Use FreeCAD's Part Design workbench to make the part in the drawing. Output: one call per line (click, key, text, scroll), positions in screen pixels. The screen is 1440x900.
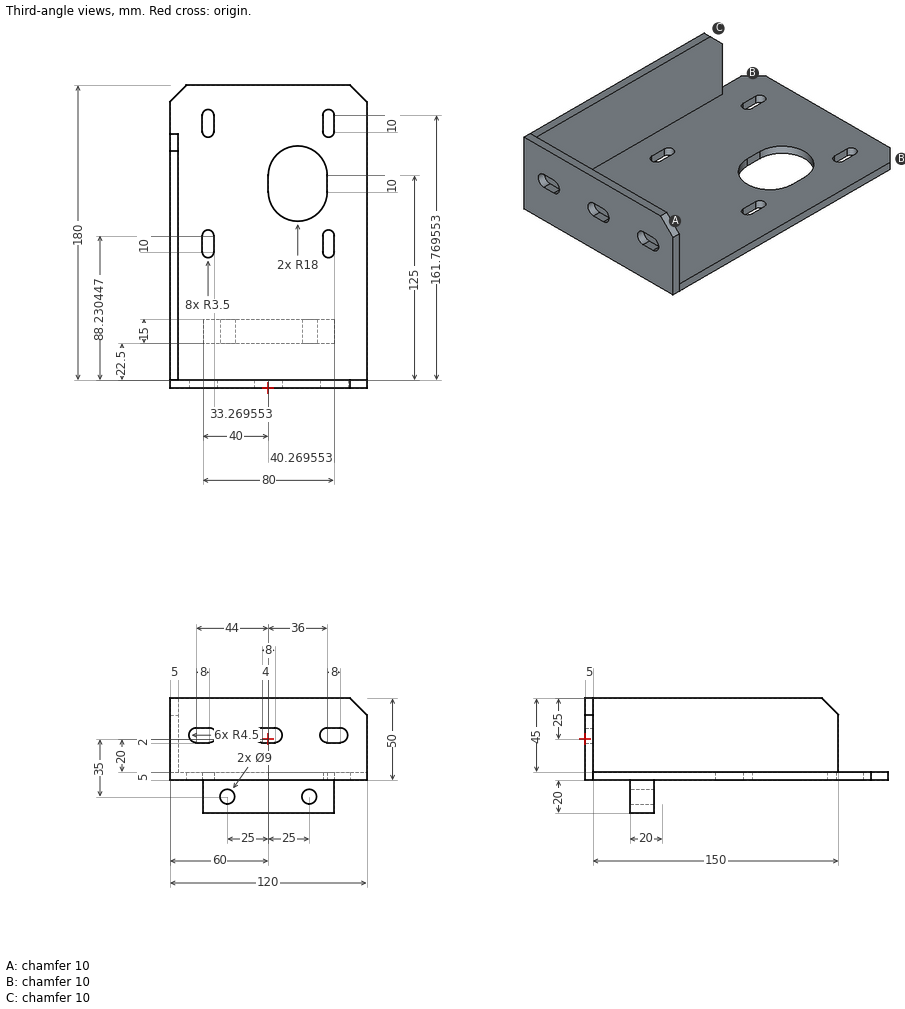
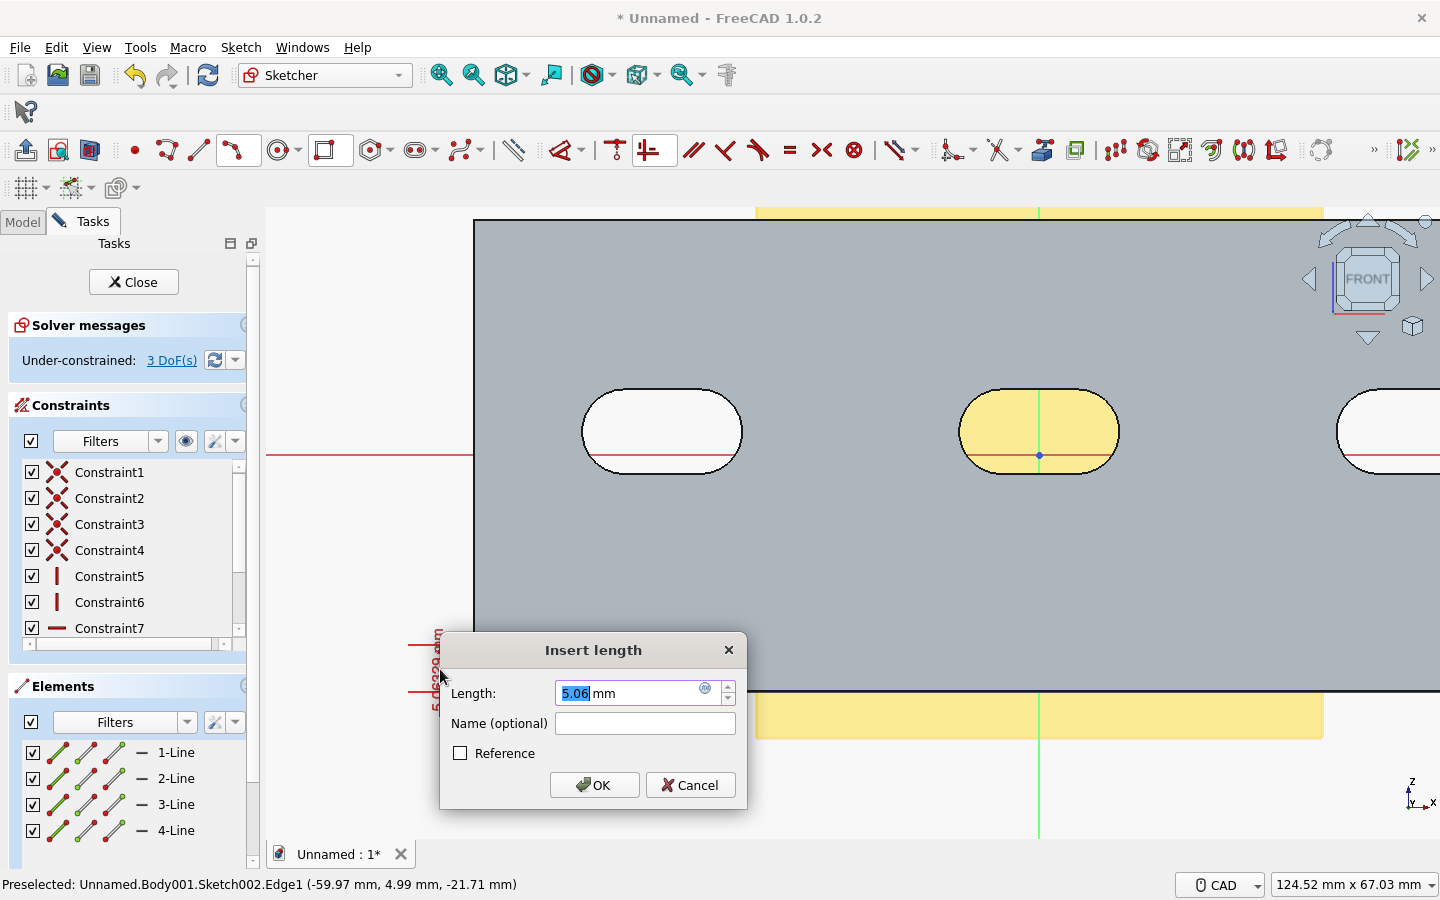
text(5)
key(Return)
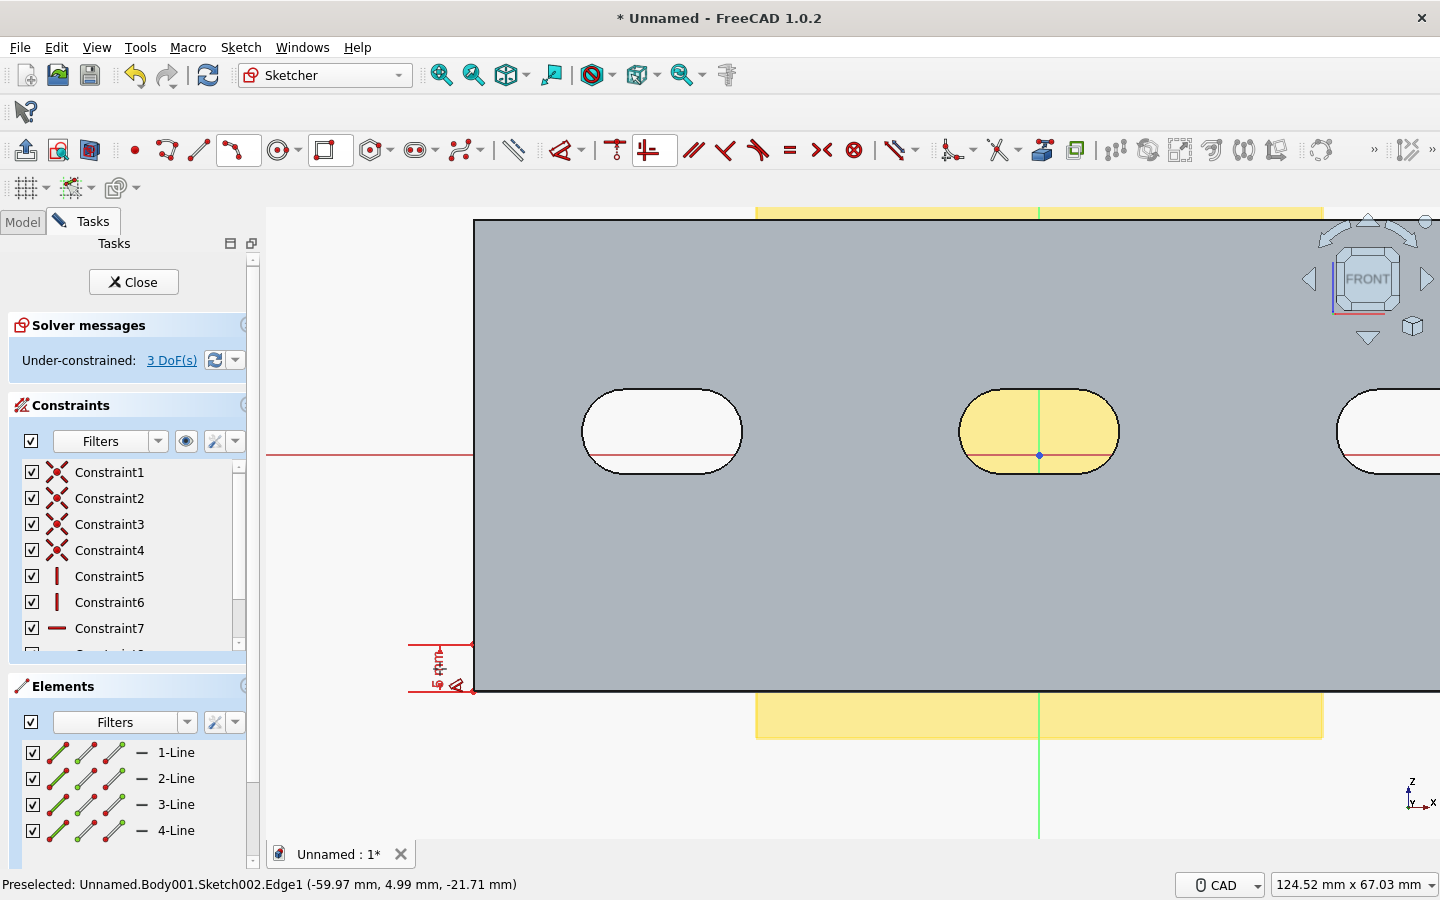
click(813, 692)
click(874, 726)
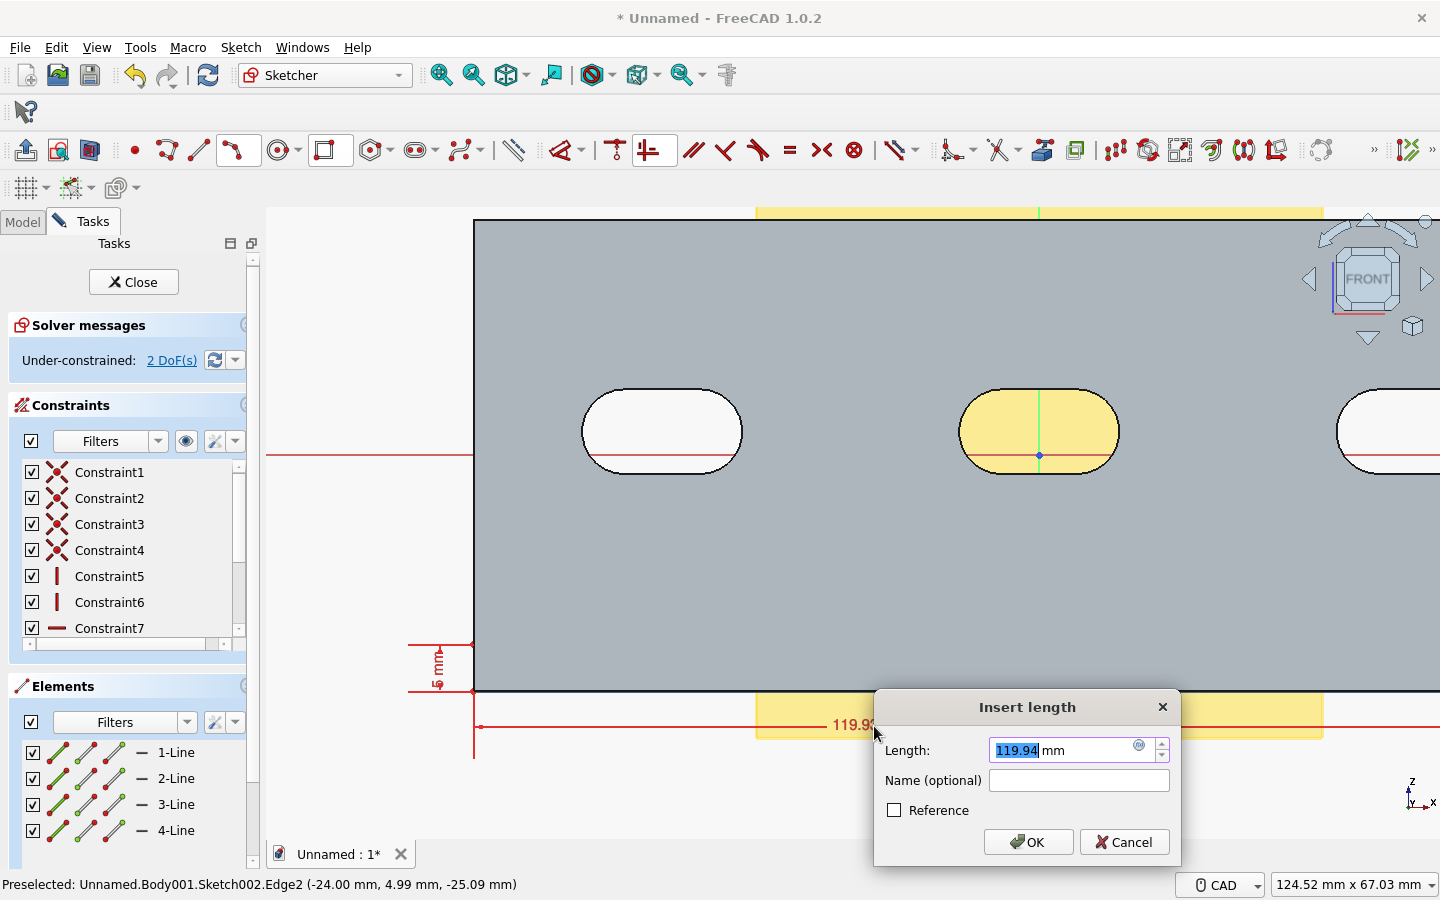
text(120)
key(Return)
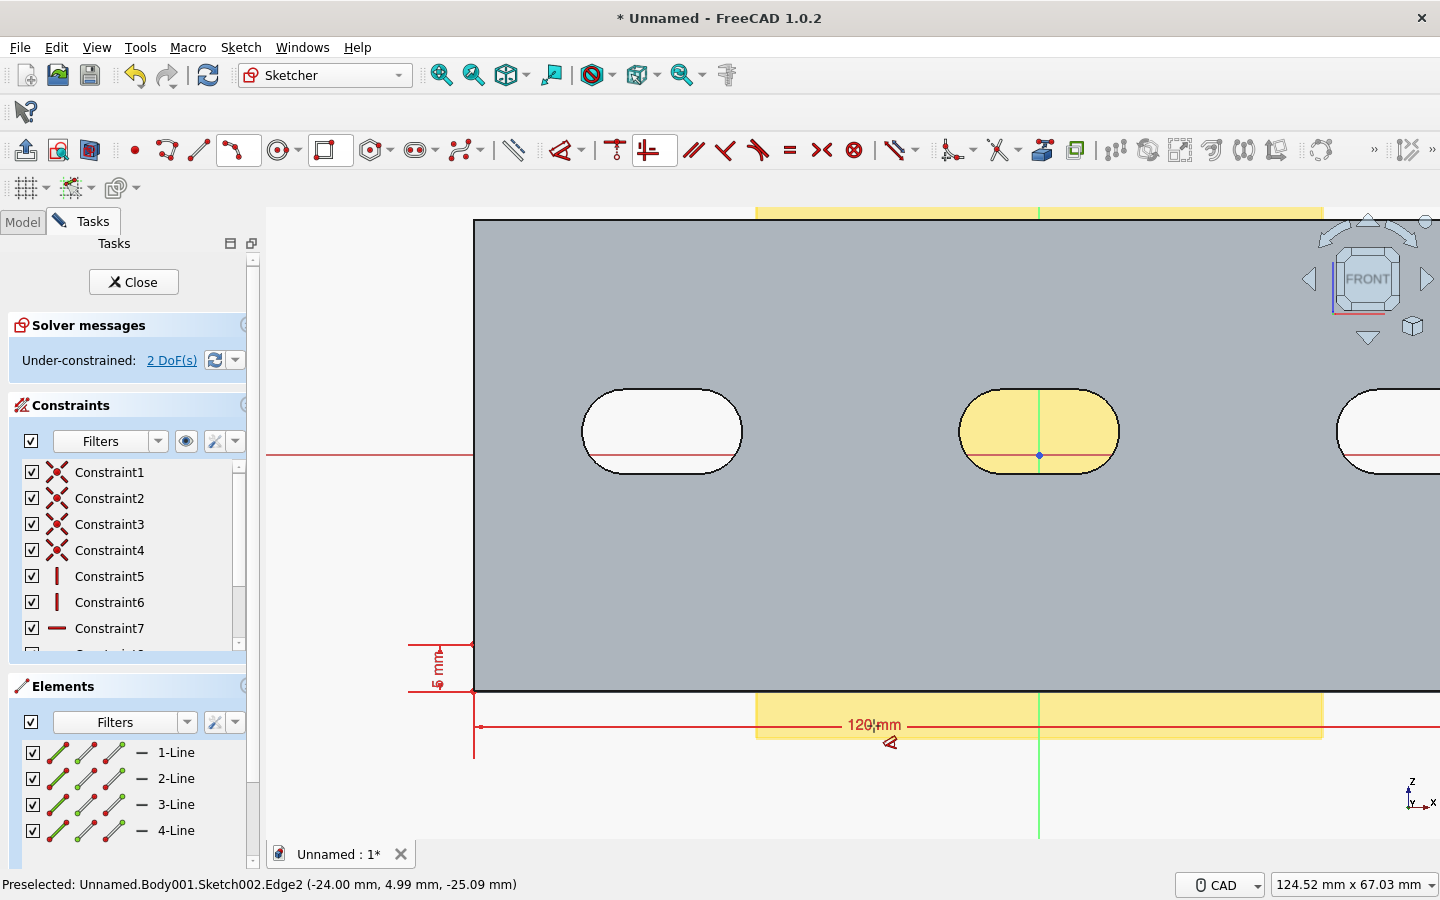
click(474, 645)
click(757, 421)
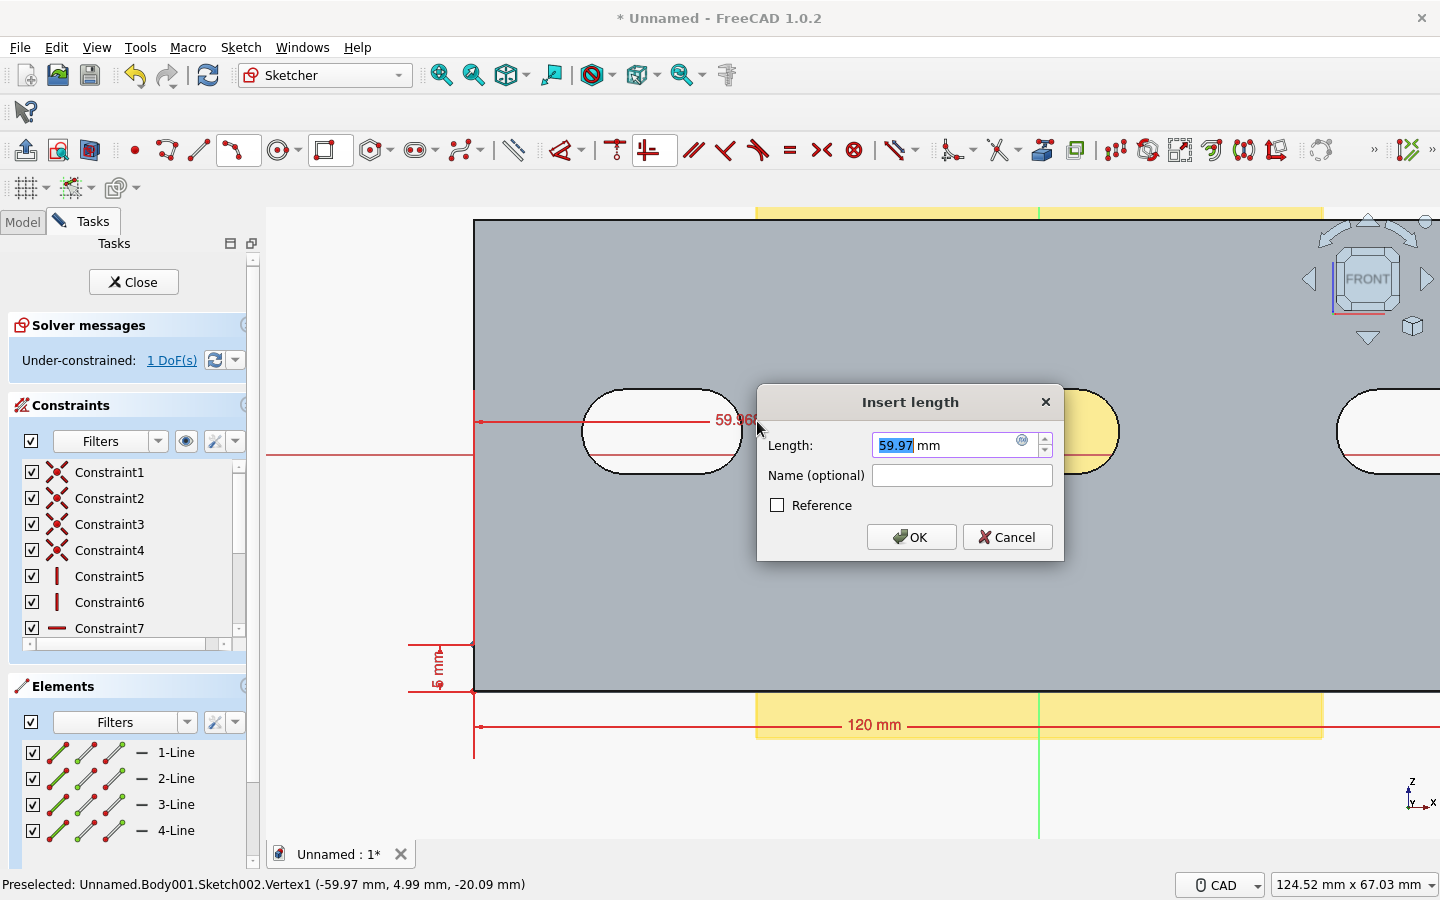
text(60)
key(Return)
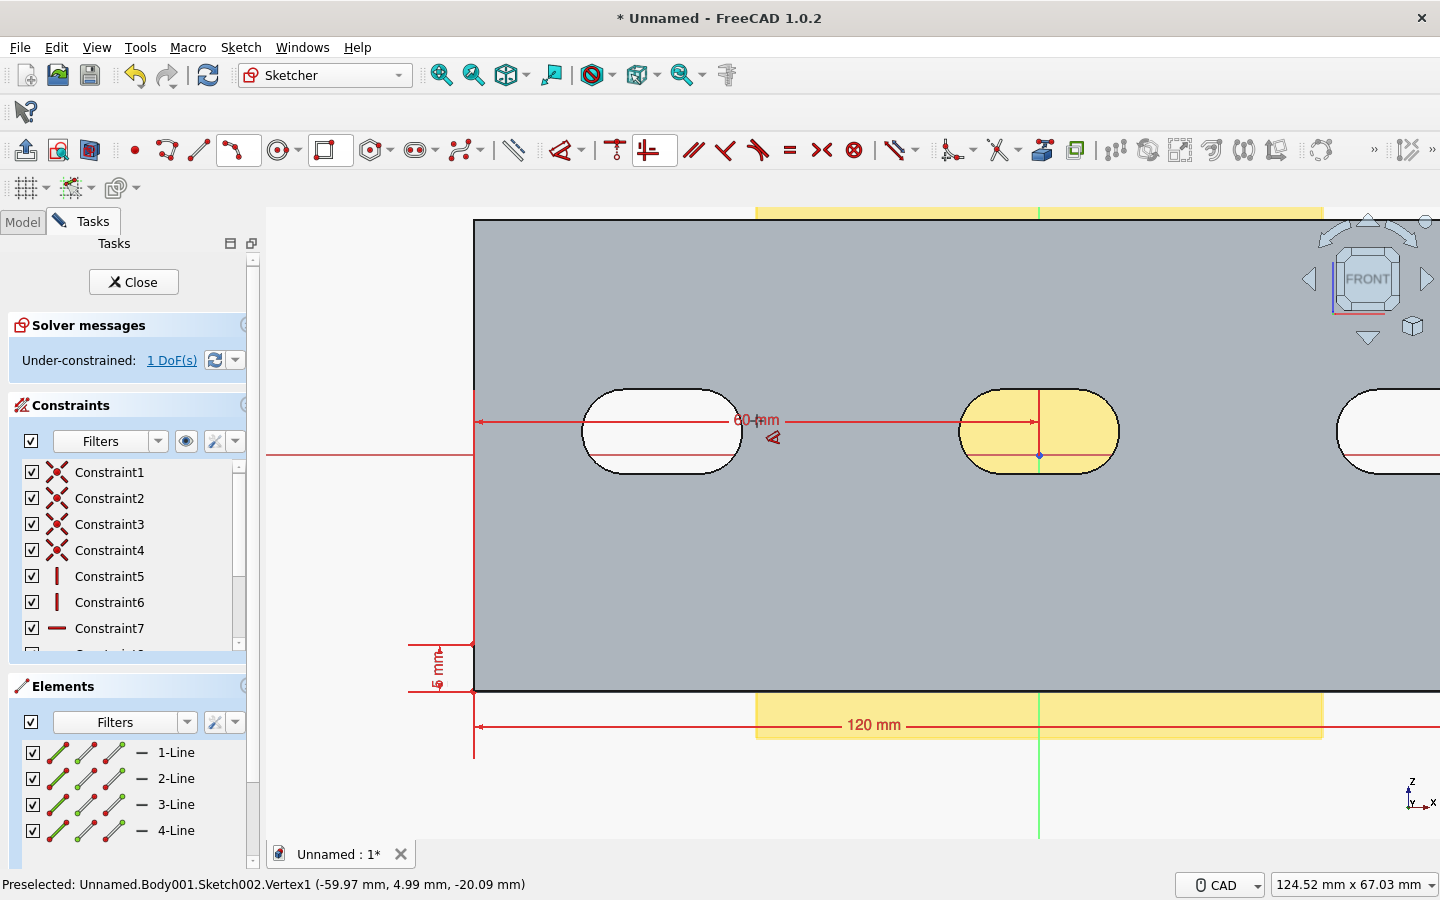
click(474, 645)
click(440, 550)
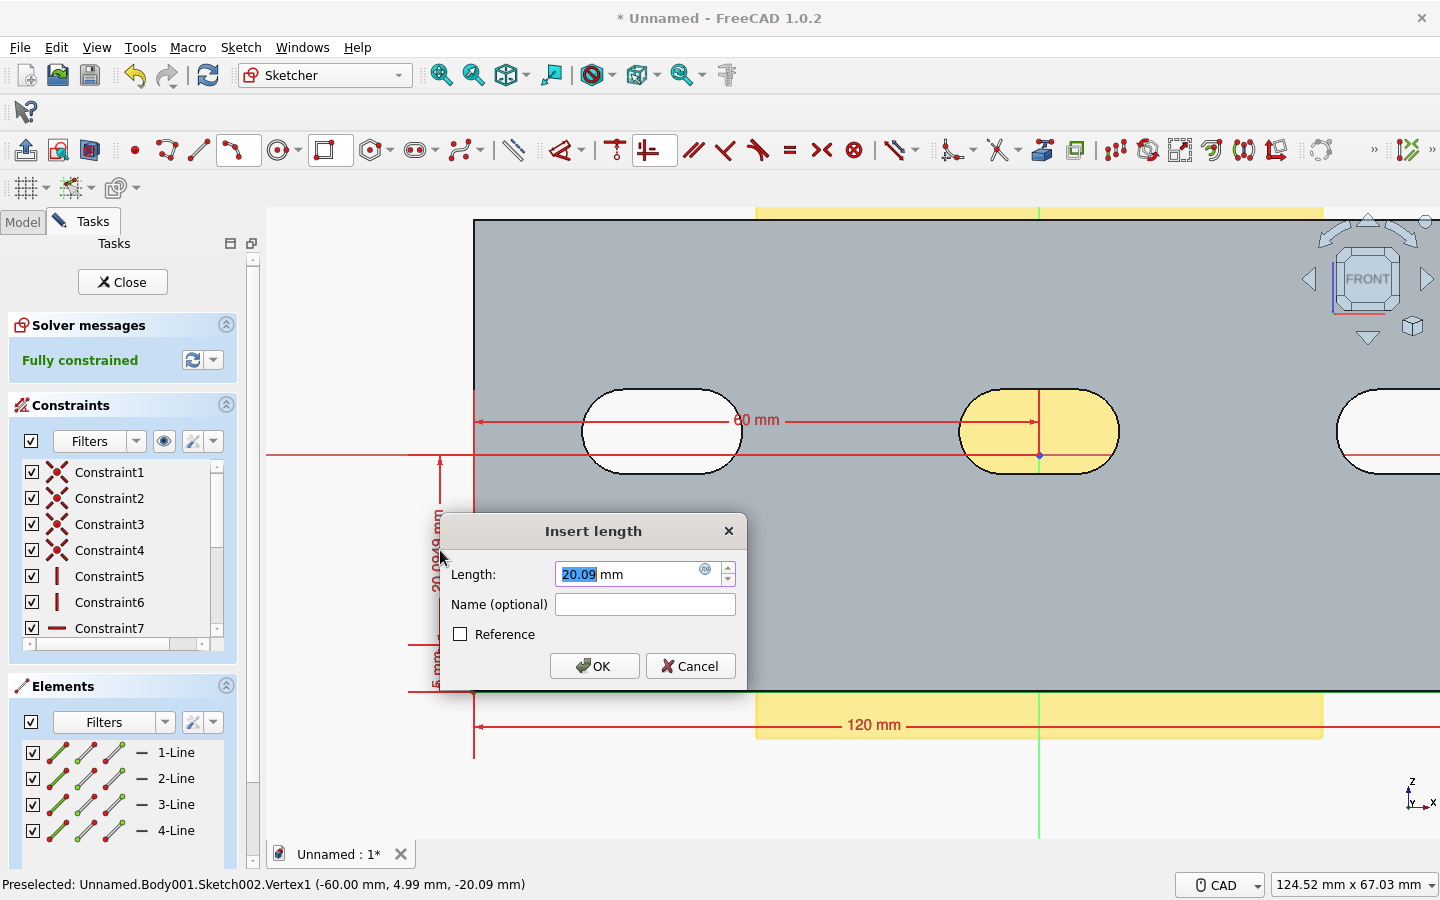
text(20)
key(Return)
key(Escape)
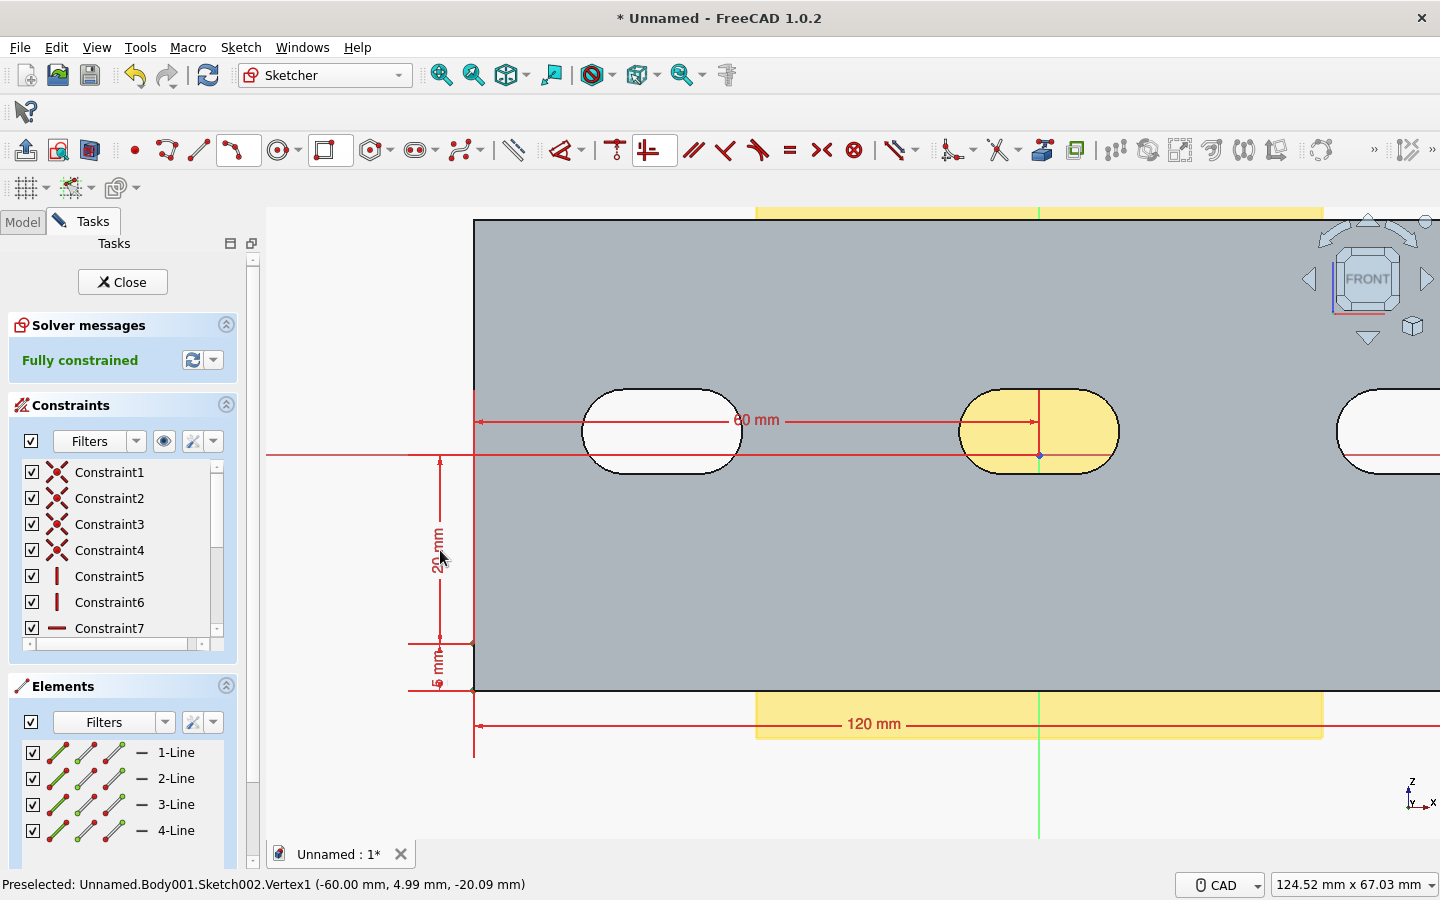
click(123, 282)